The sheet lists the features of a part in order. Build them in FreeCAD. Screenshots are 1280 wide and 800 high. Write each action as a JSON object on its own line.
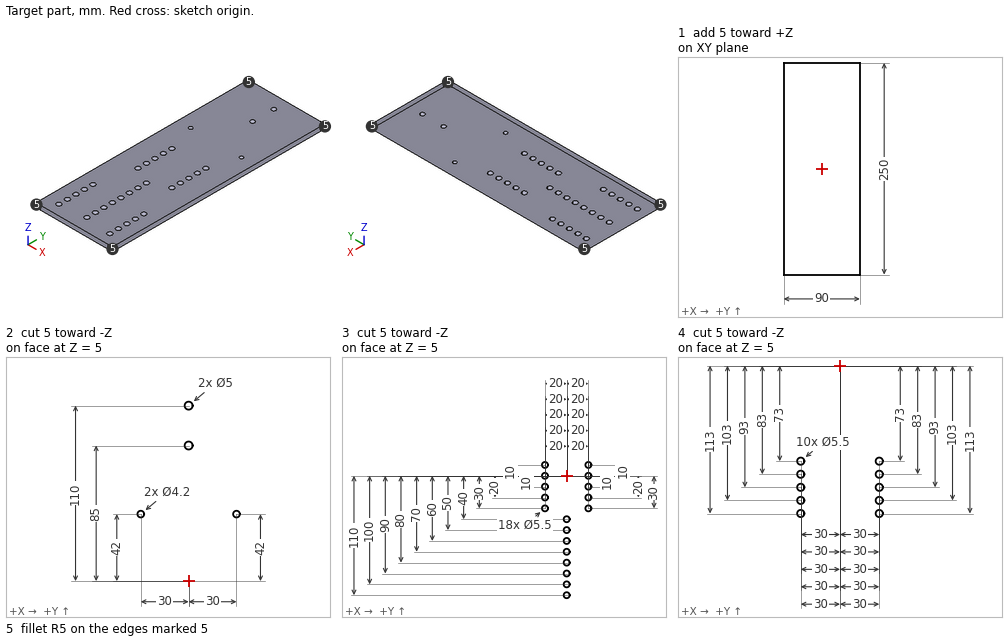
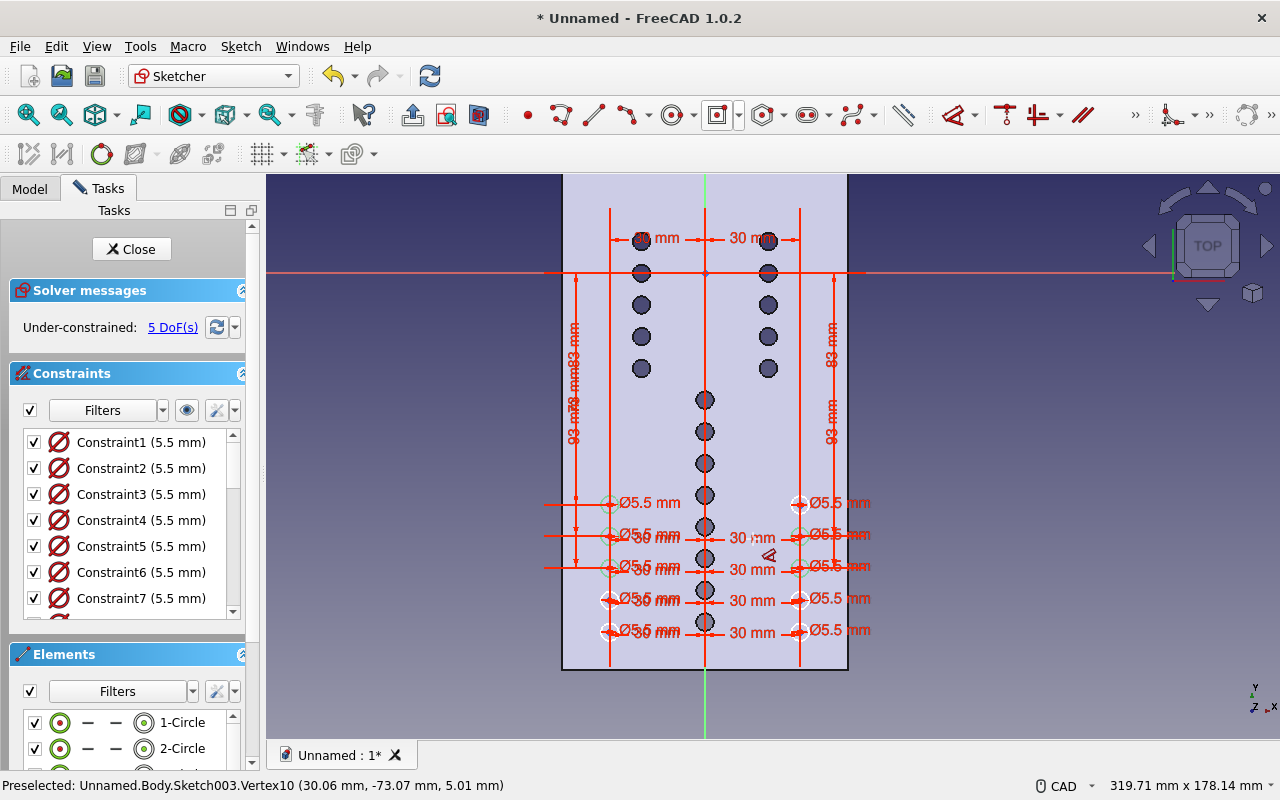
{"action": "left_click", "coordinate": [800, 505]}
{"action": "left_click", "coordinate": [834, 389]}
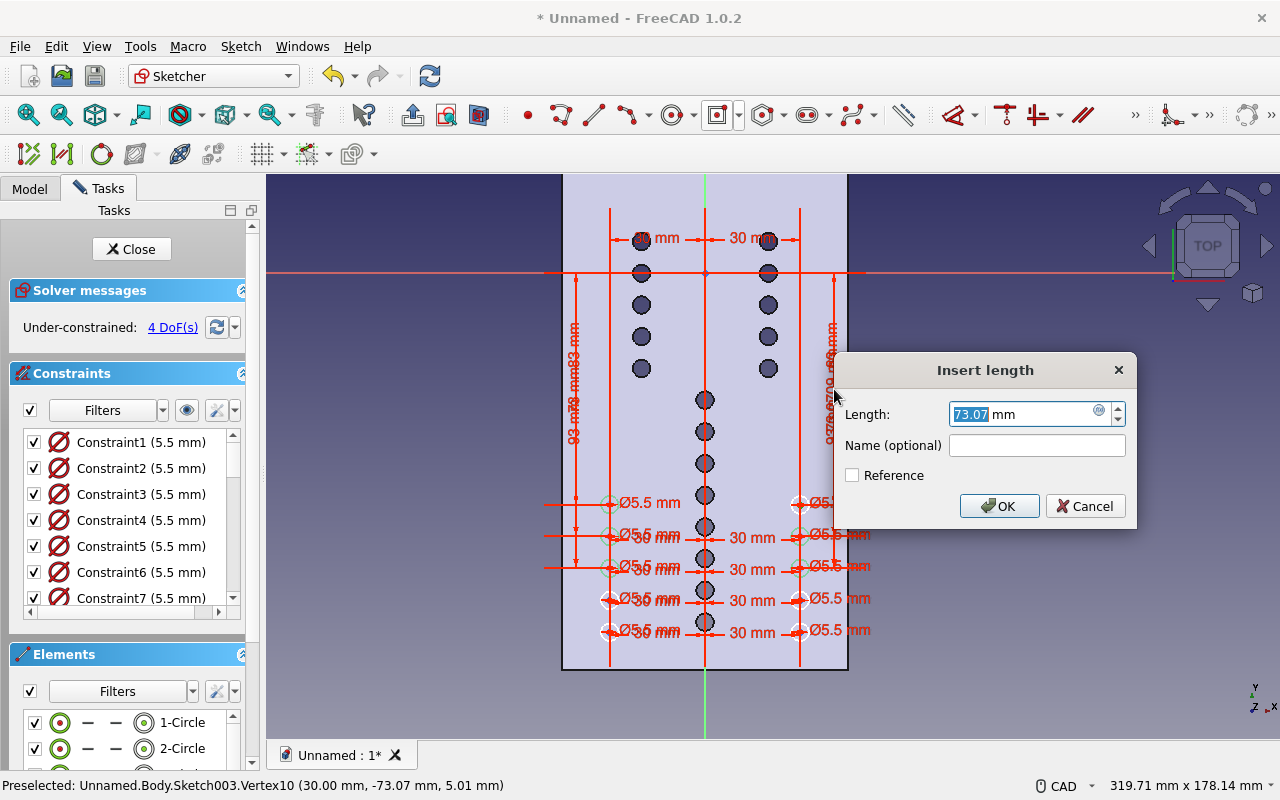
{"action": "type", "text": "73"}
{"action": "key", "text": "Return"}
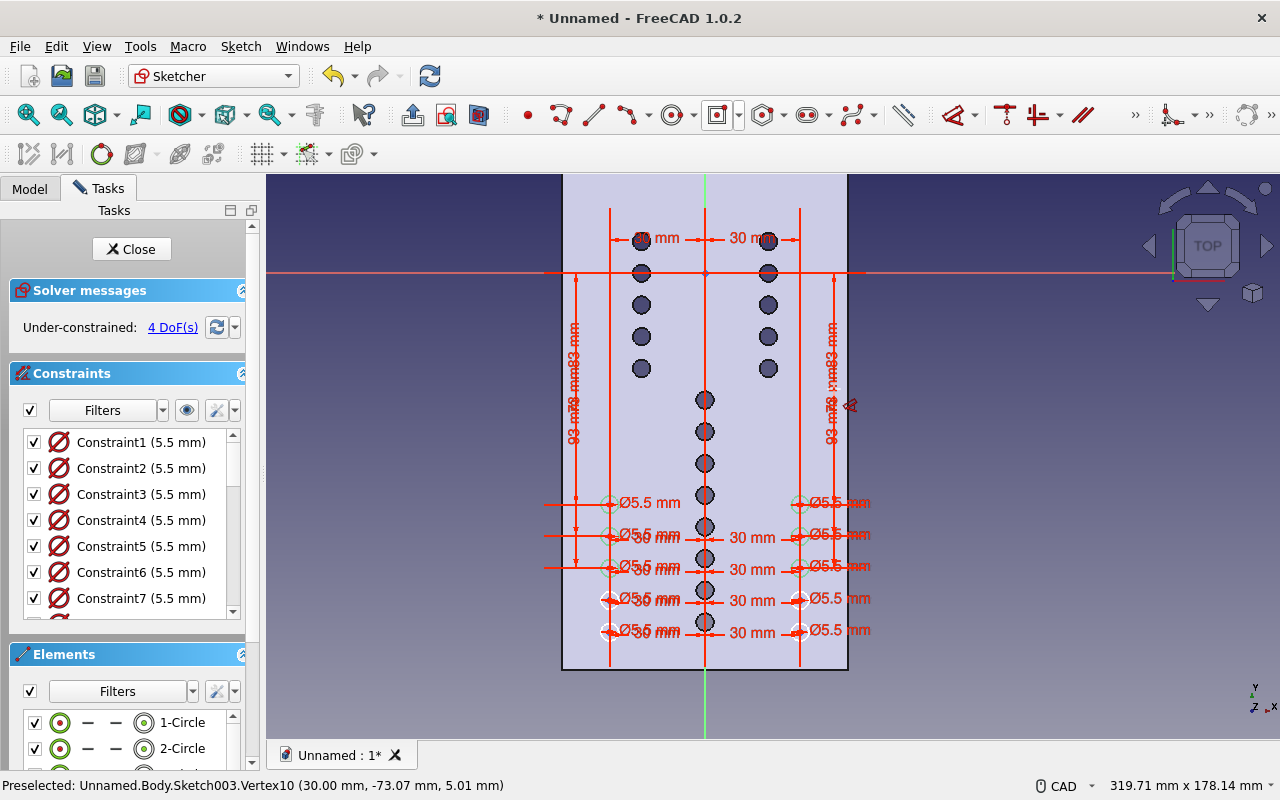
{"action": "left_click", "coordinate": [610, 632]}
{"action": "left_click", "coordinate": [576, 453]}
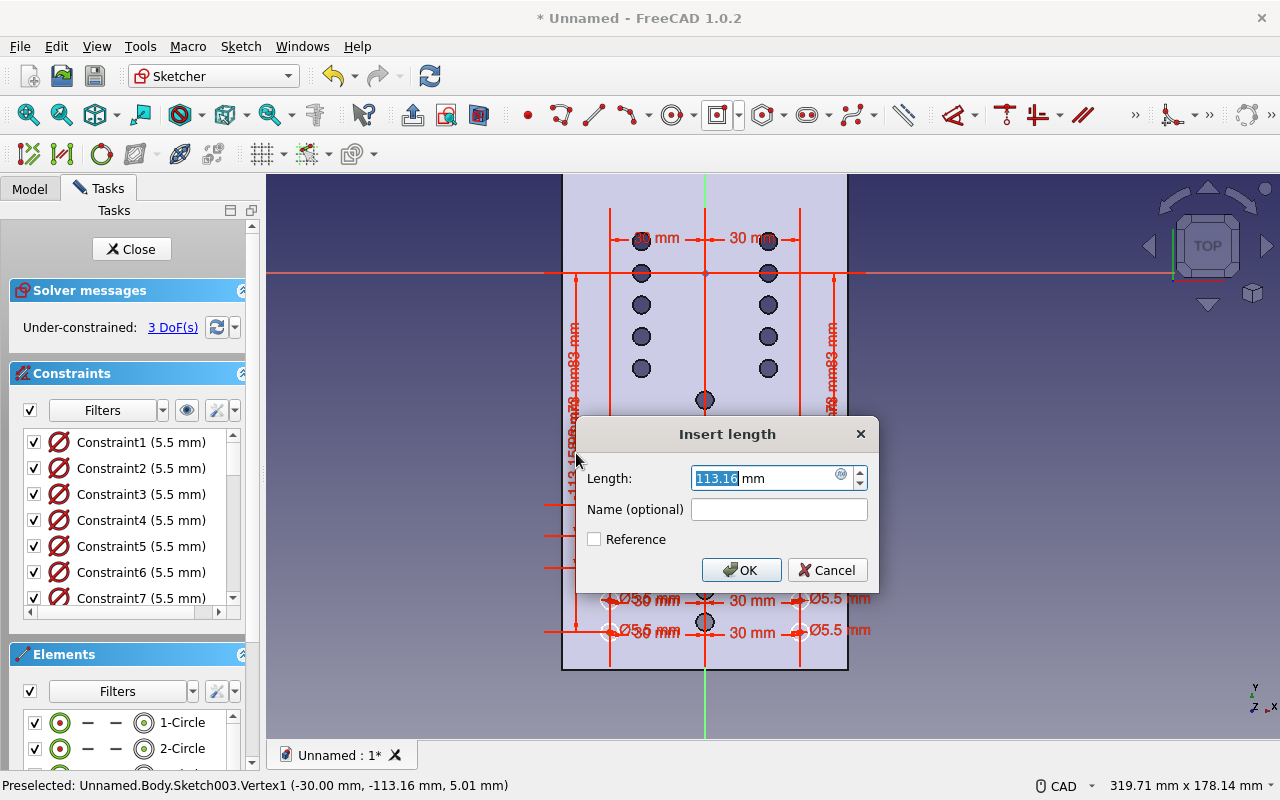
{"action": "type", "text": "113"}
{"action": "key", "text": "Return"}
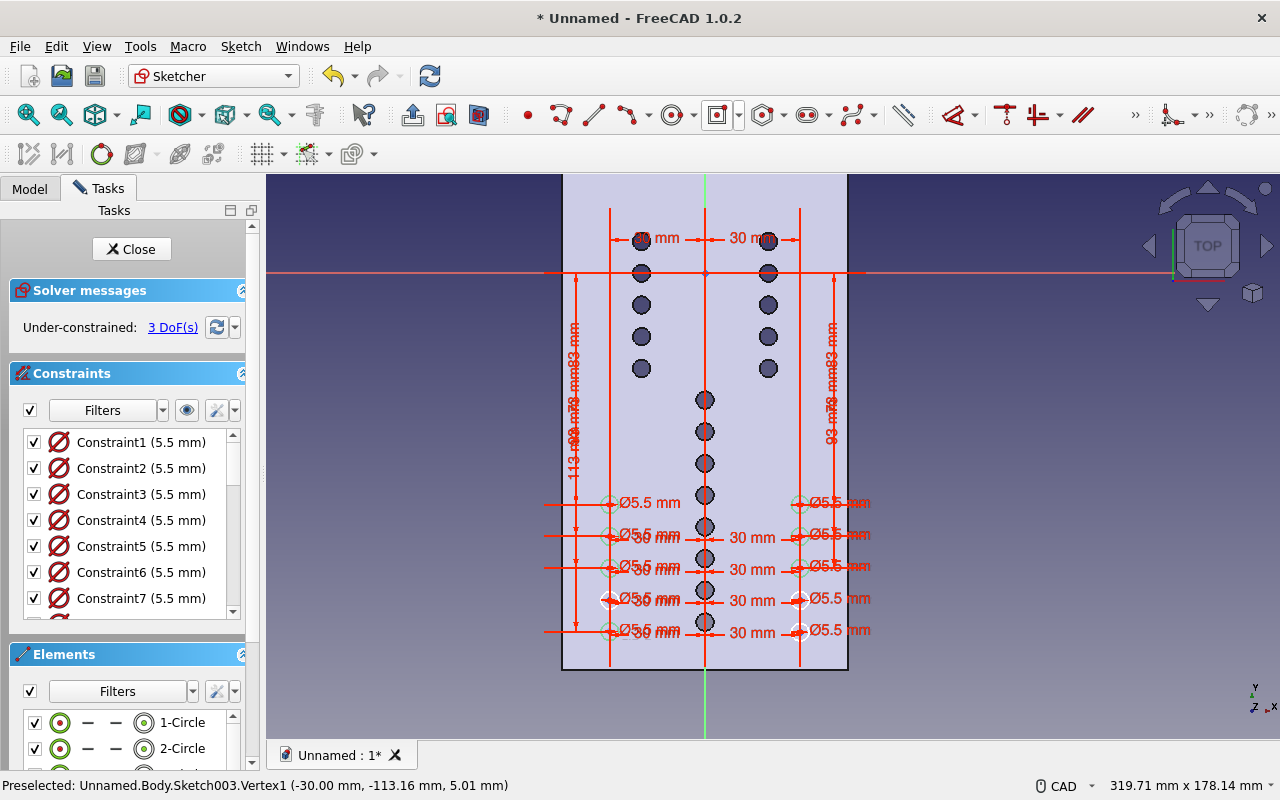
{"action": "left_click", "coordinate": [800, 632]}
{"action": "left_click", "coordinate": [834, 453]}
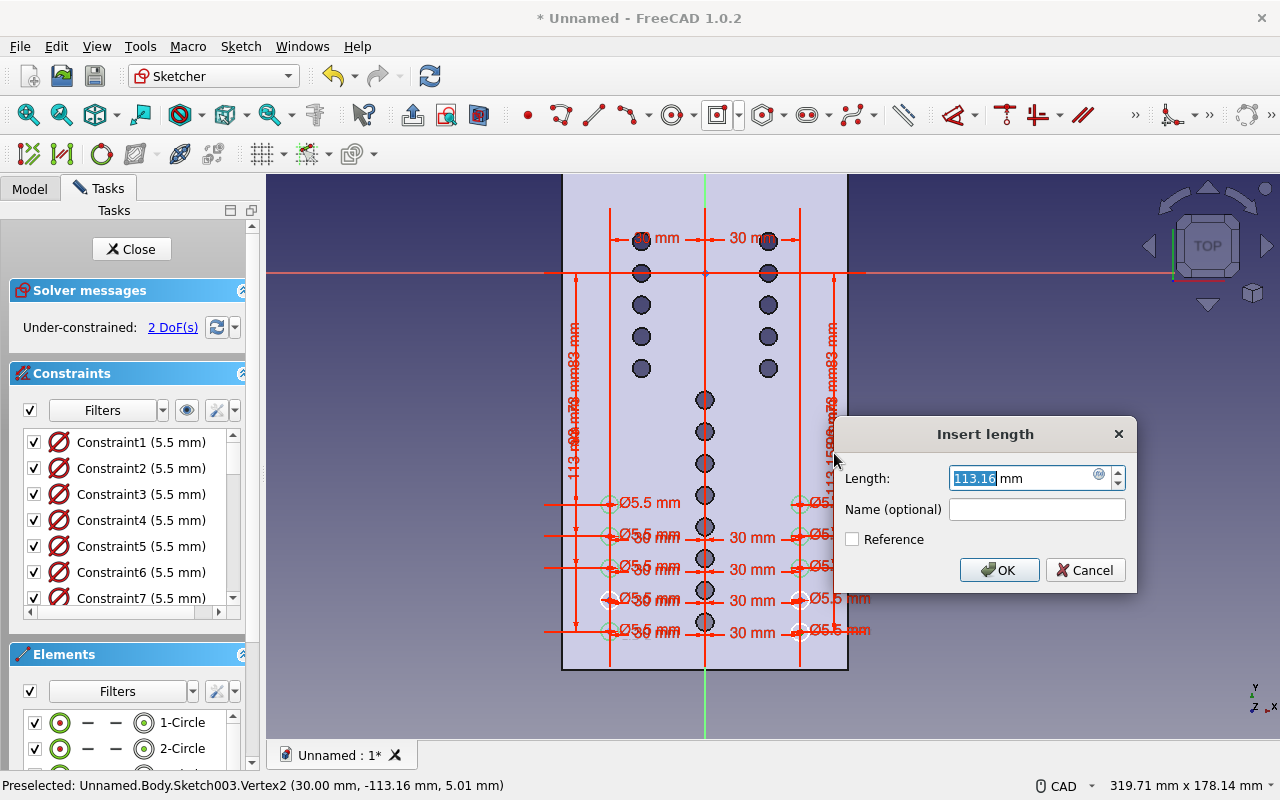
{"action": "type", "text": "113"}
{"action": "key", "text": "Return"}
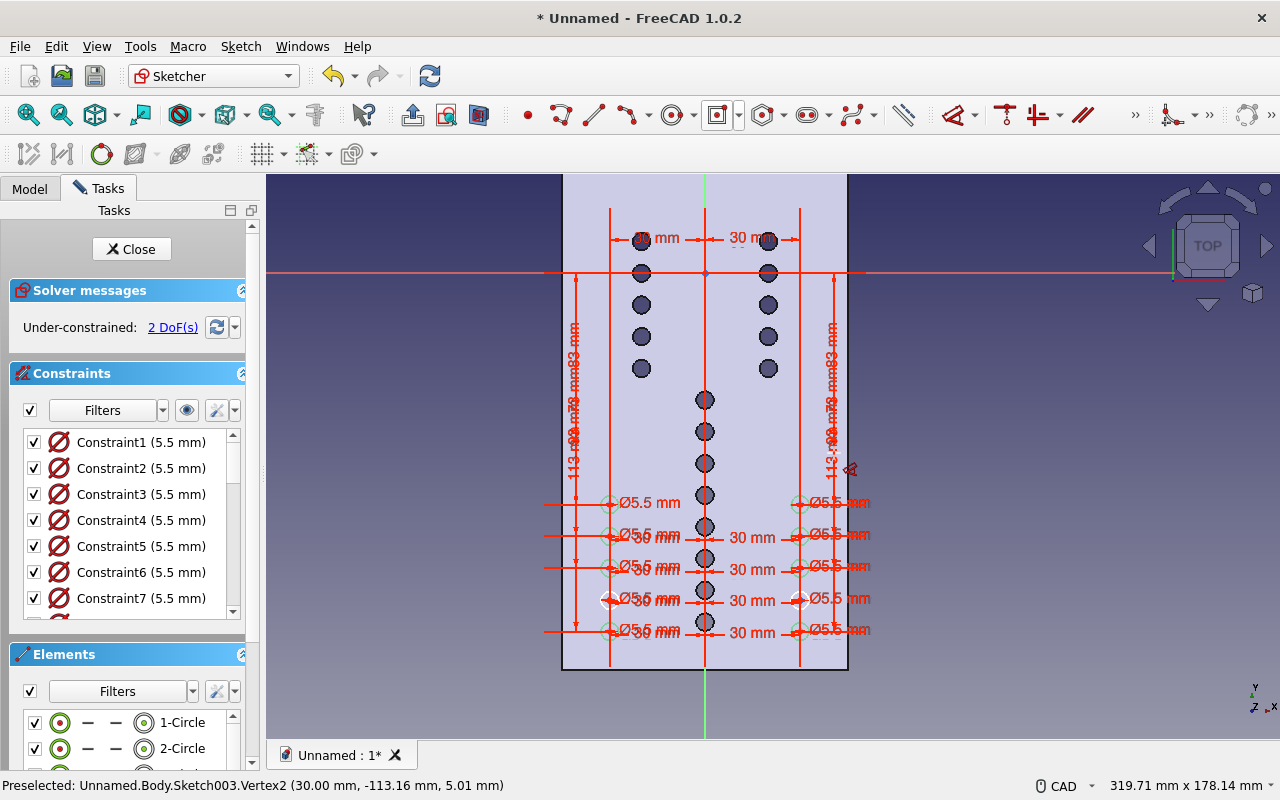
{"action": "left_click", "coordinate": [610, 600]}
{"action": "left_click", "coordinate": [576, 512]}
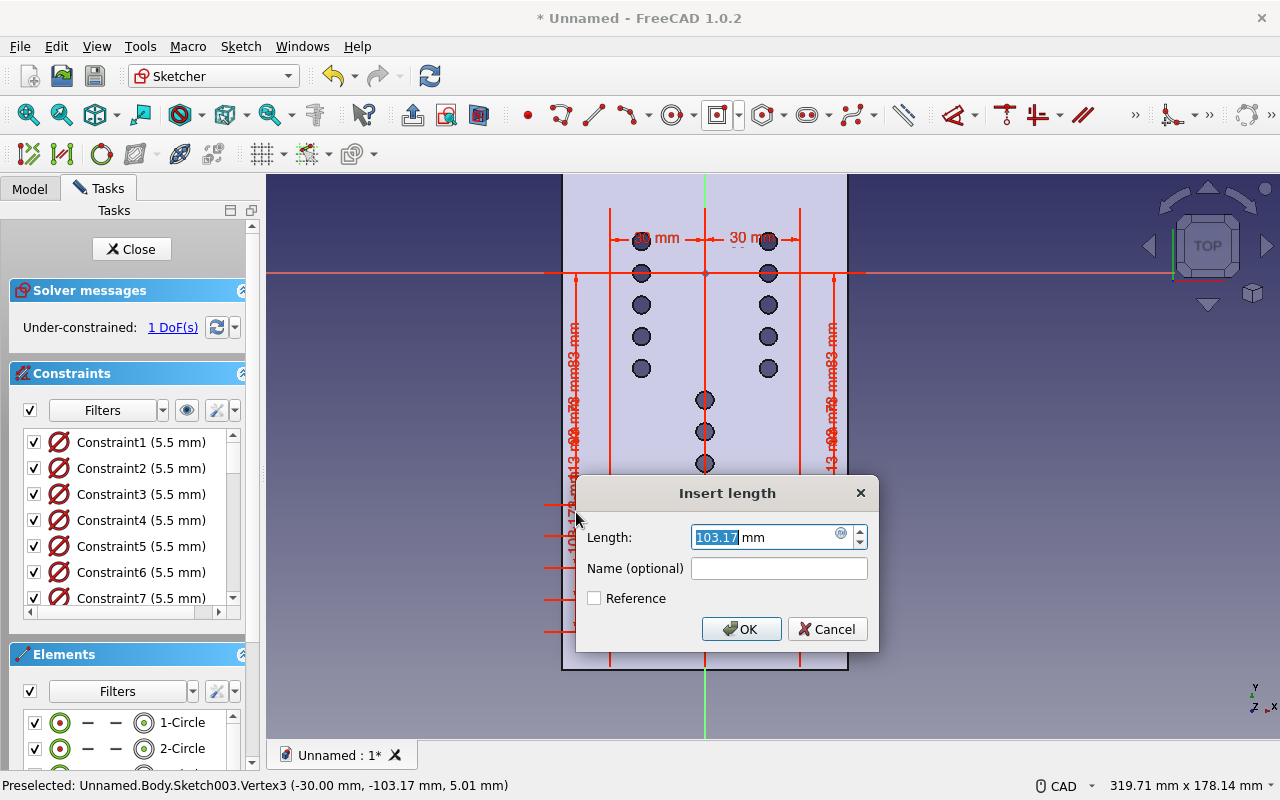
{"action": "type", "text": "103"}
{"action": "key", "text": "Return"}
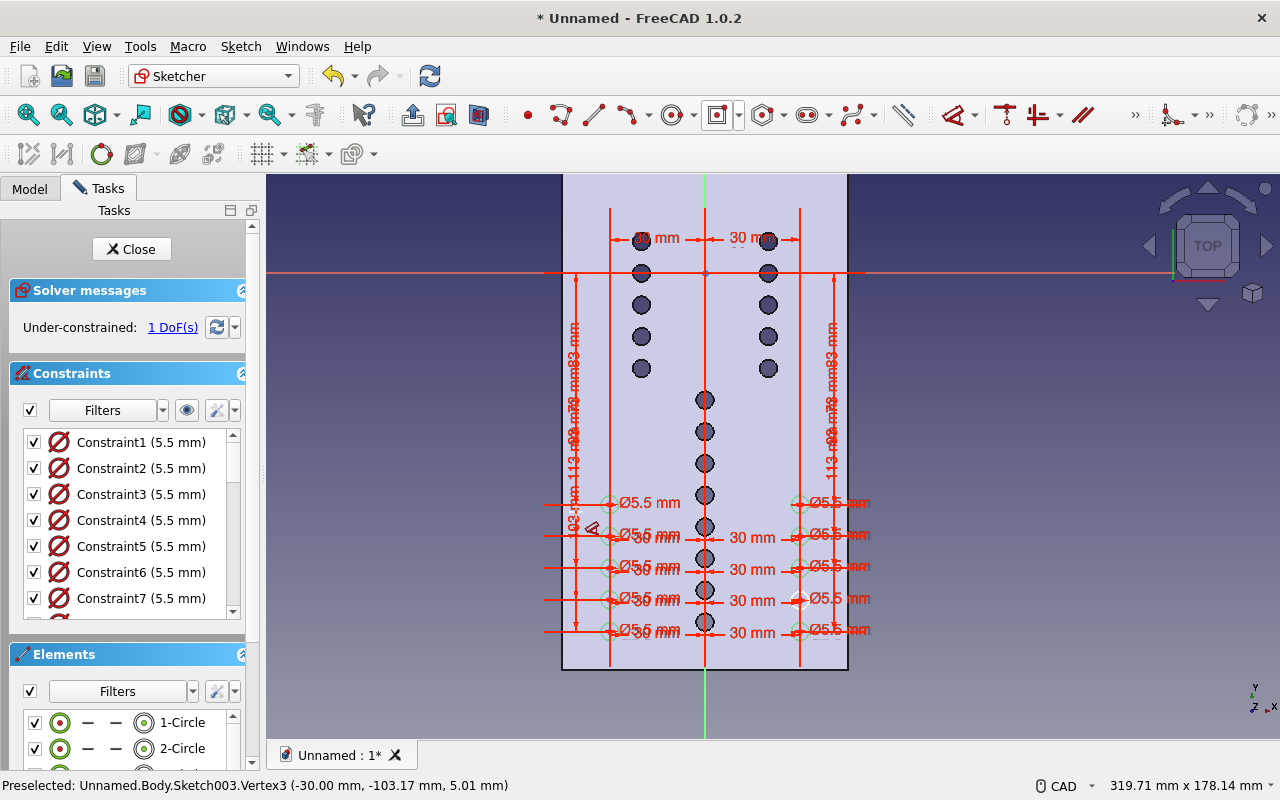
{"action": "left_click", "coordinate": [800, 600]}
{"action": "left_click", "coordinate": [834, 512]}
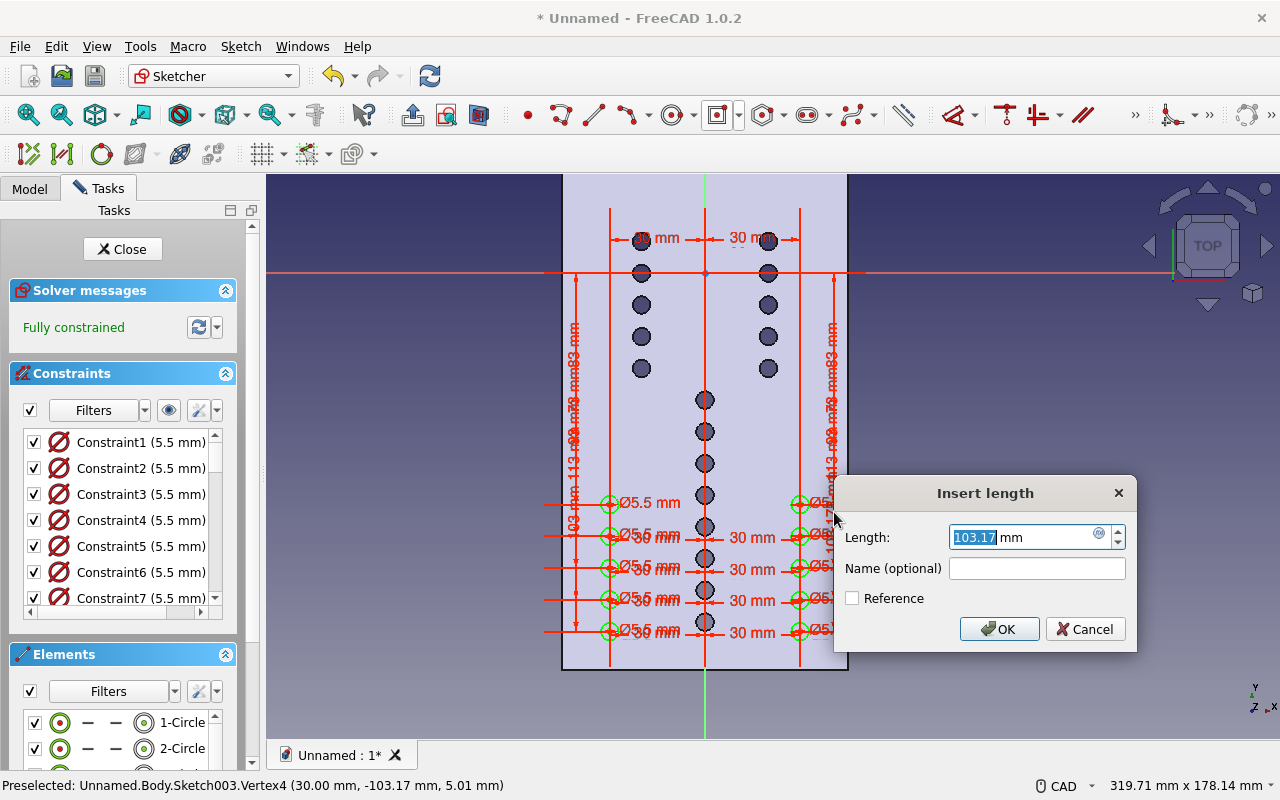
{"action": "type", "text": "103"}
{"action": "key", "text": "Return"}
{"action": "key", "text": "Escape"}